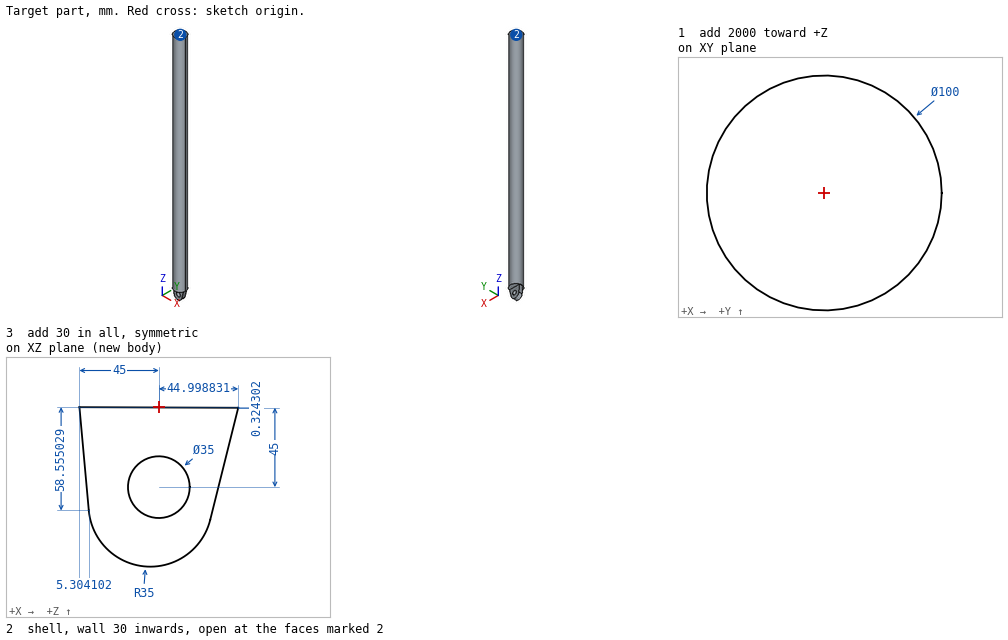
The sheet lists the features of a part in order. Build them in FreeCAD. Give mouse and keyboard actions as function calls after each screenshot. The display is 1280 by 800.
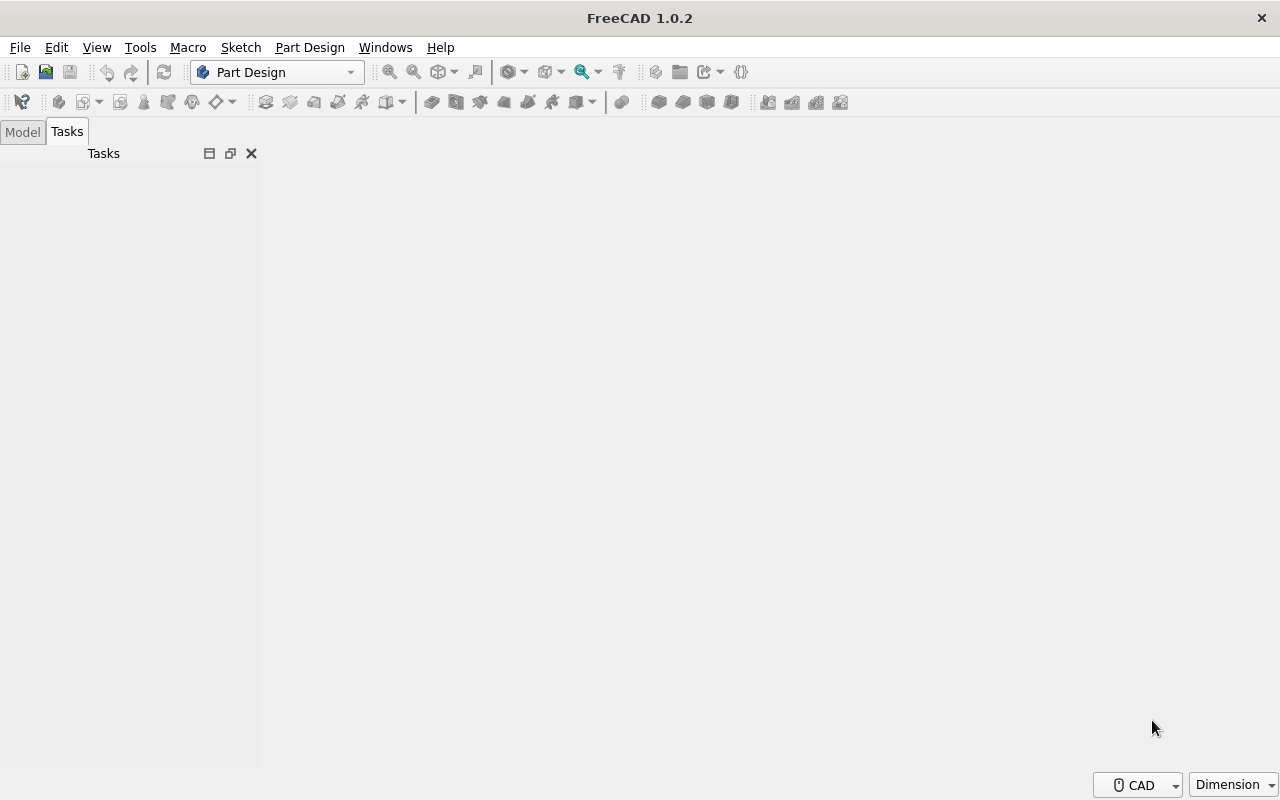
key(ctrl+n)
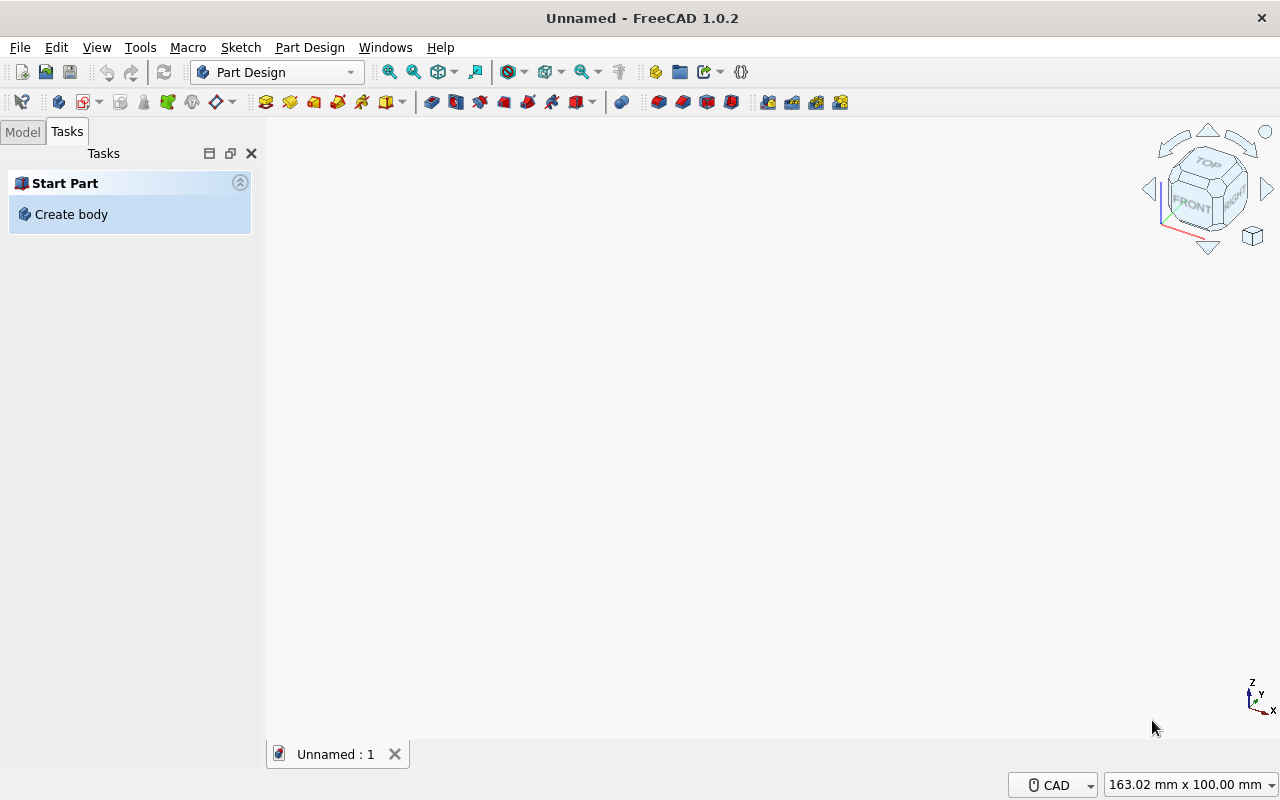
click(84, 102)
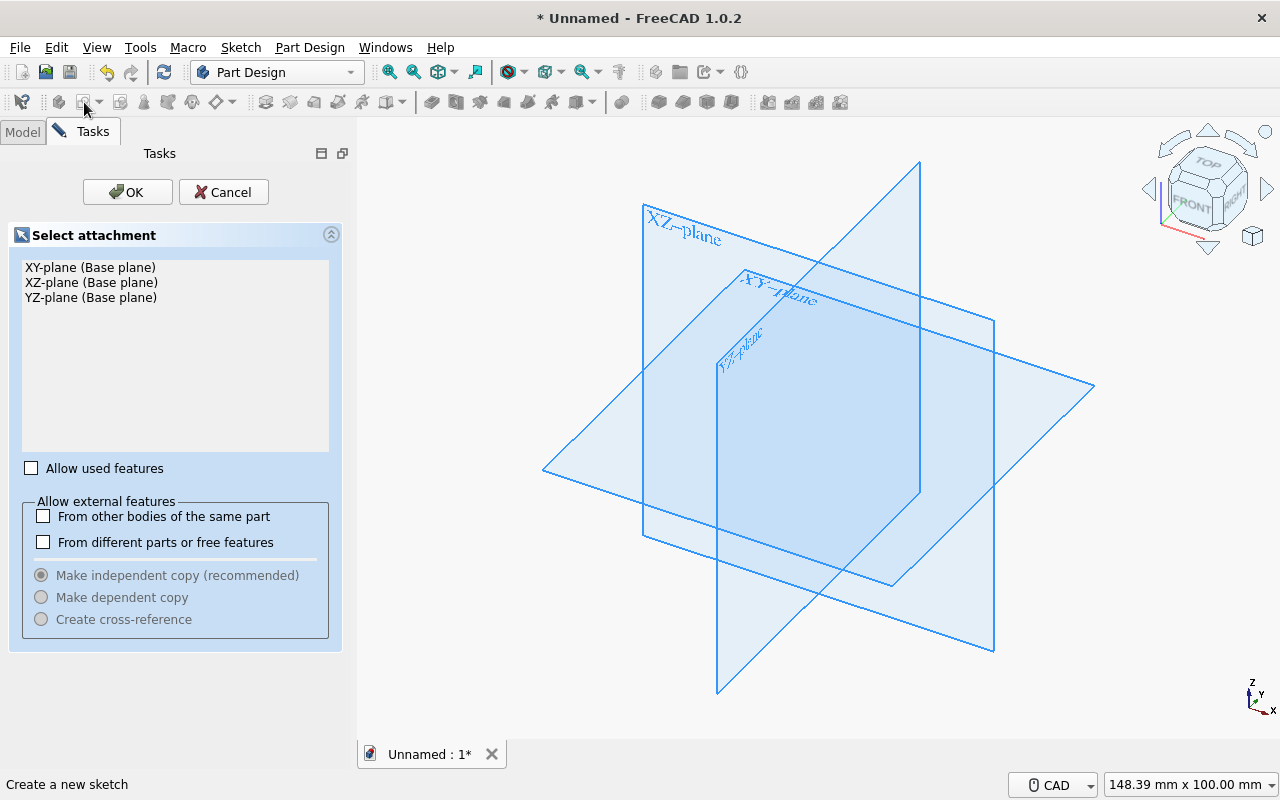
click(82, 268)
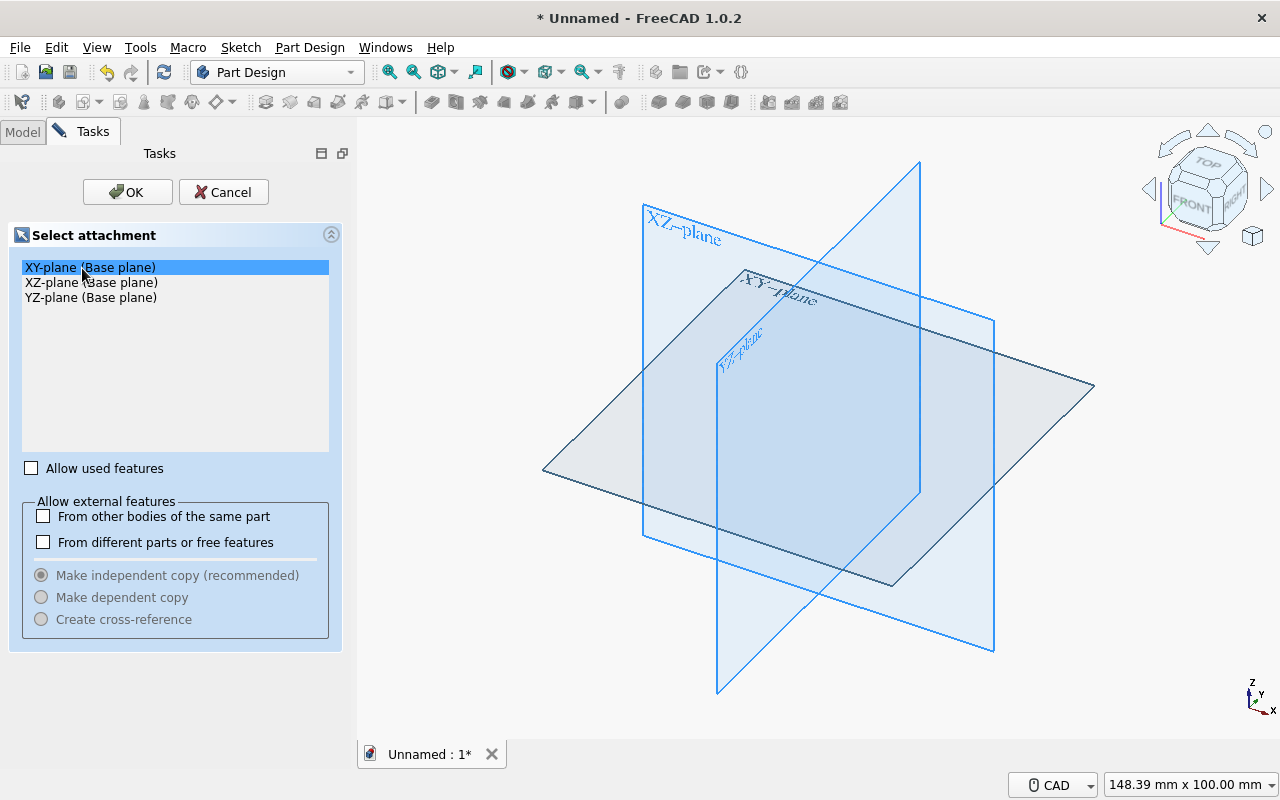
click(128, 192)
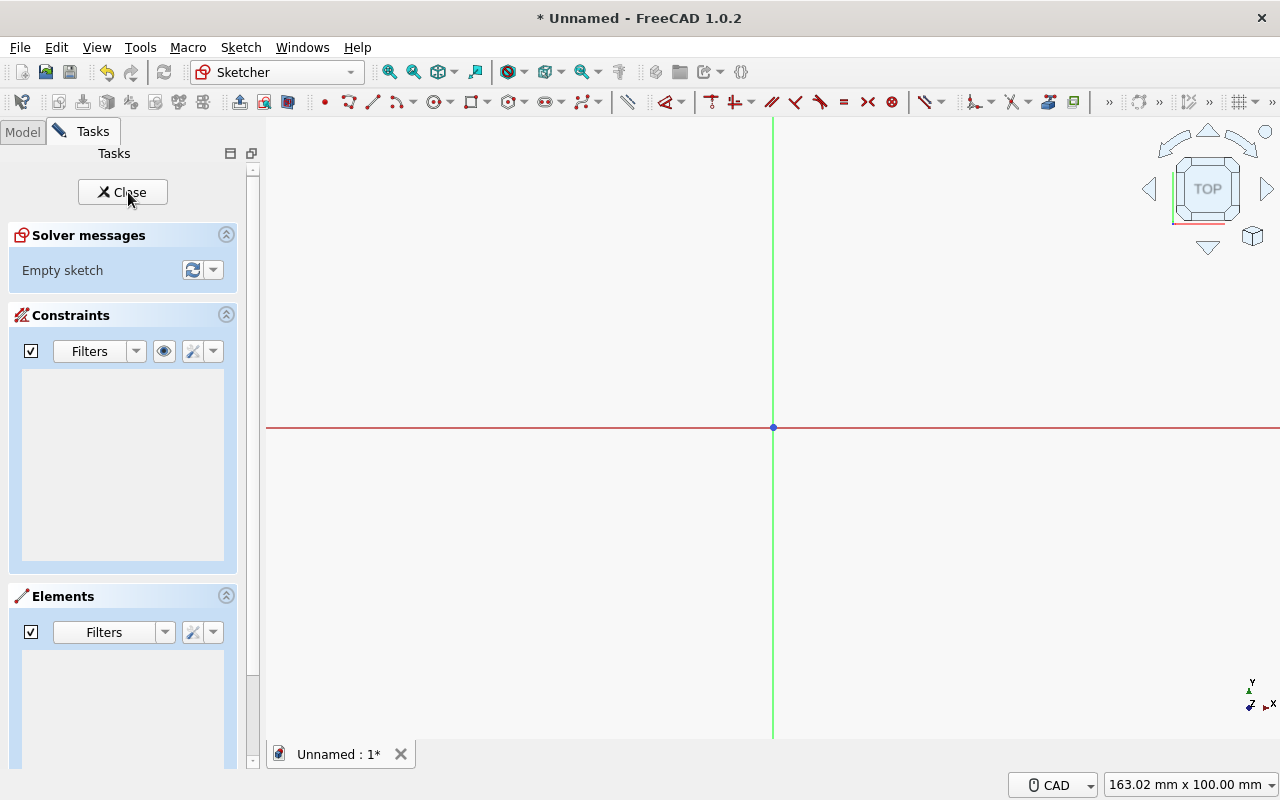
scroll(565, 428, down, 2)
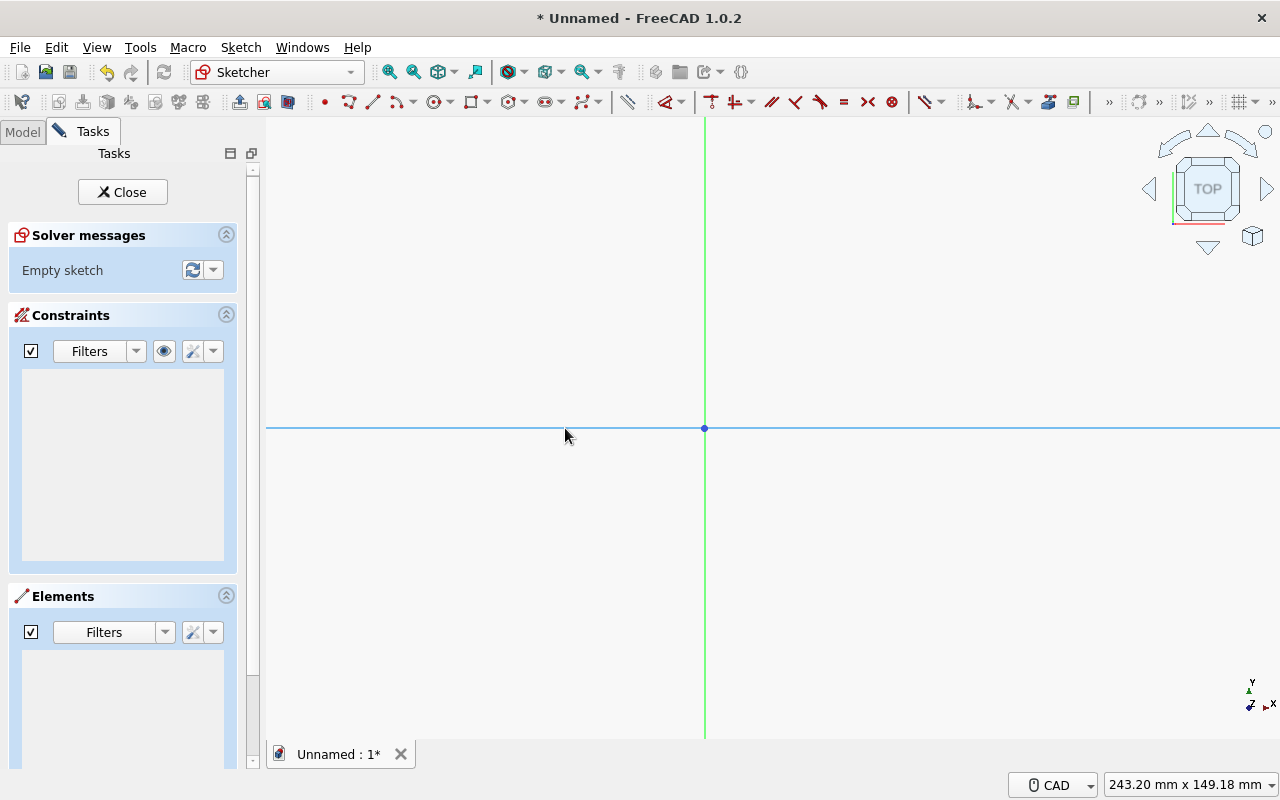
key(g)
key(c)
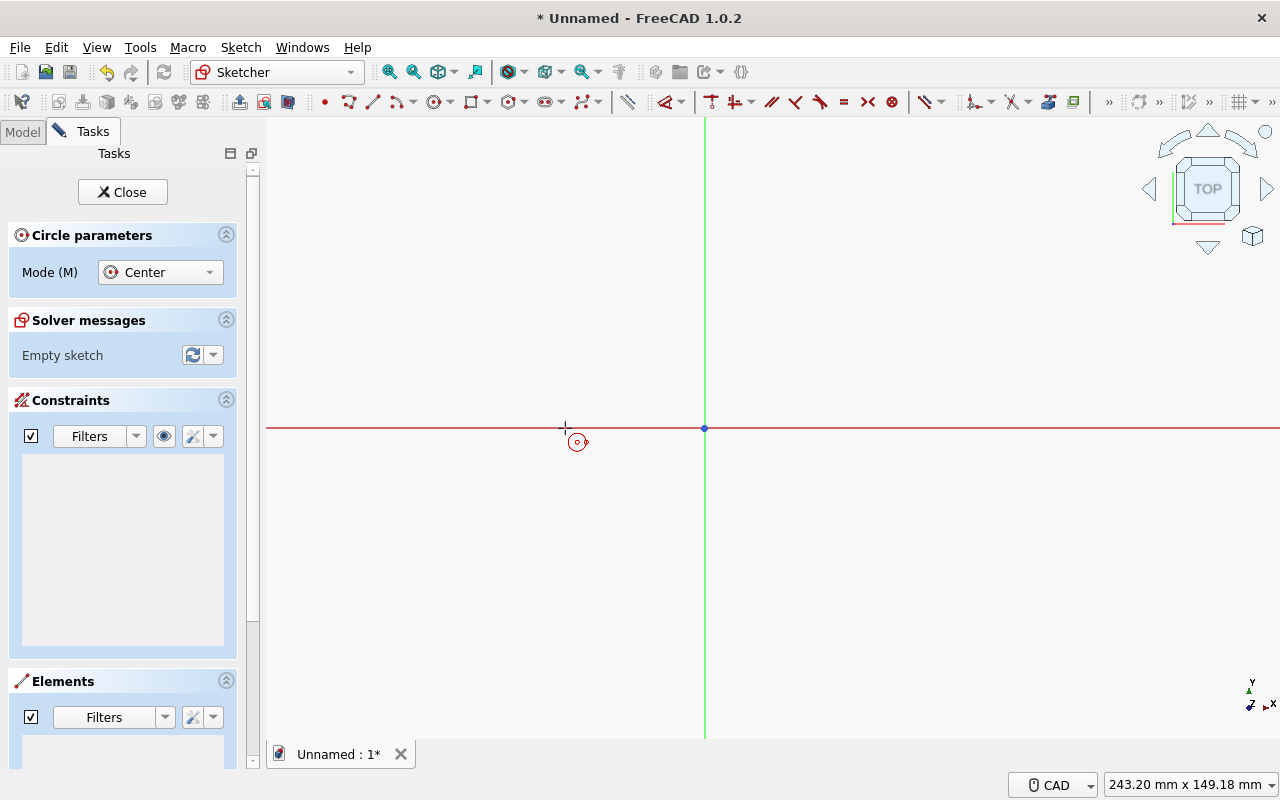
click(705, 428)
click(852, 281)
key(Escape)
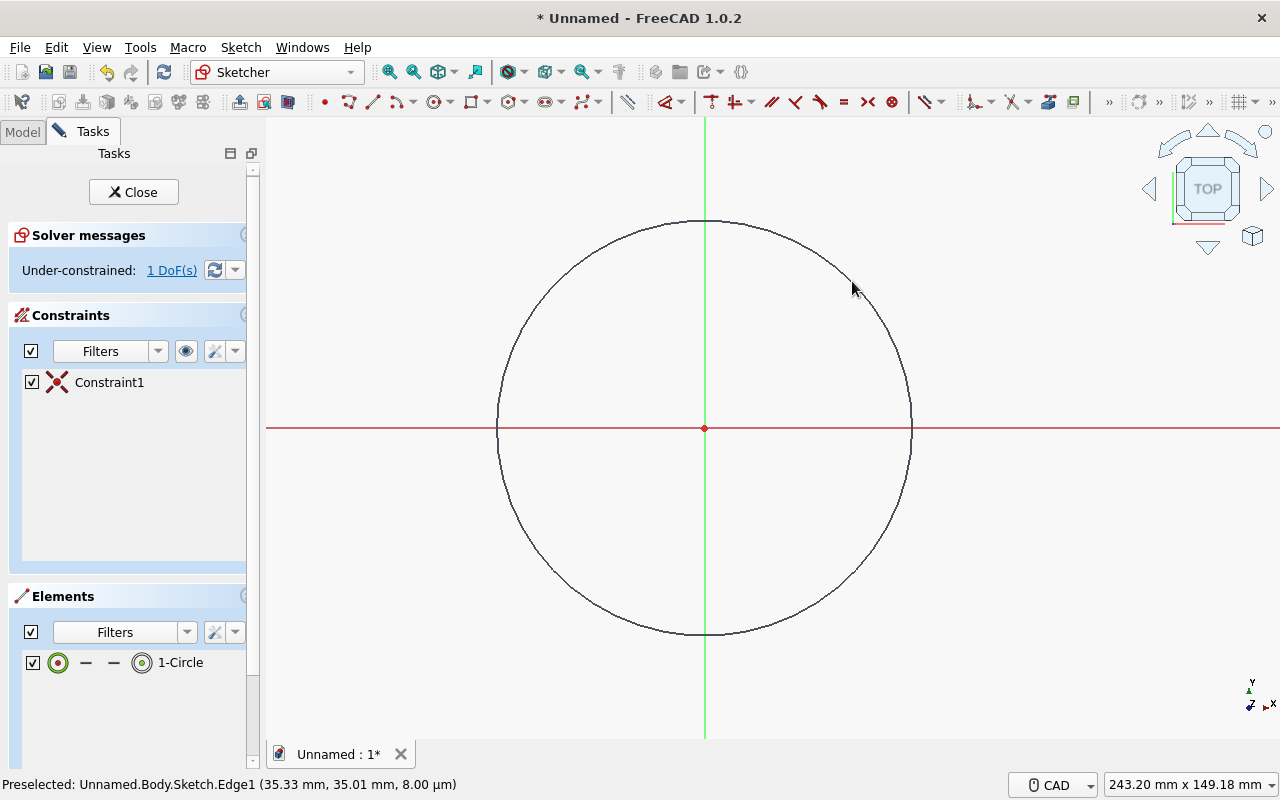
key(d)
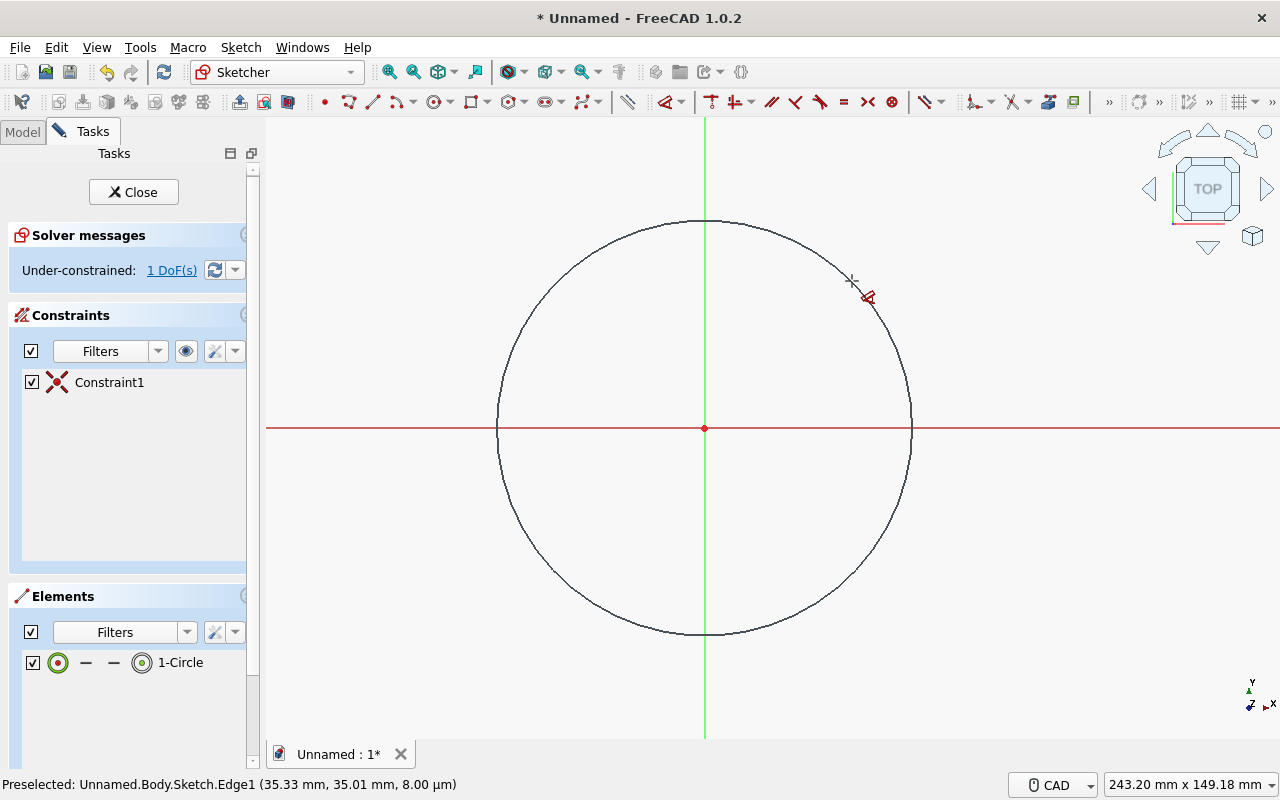
click(851, 281)
click(874, 258)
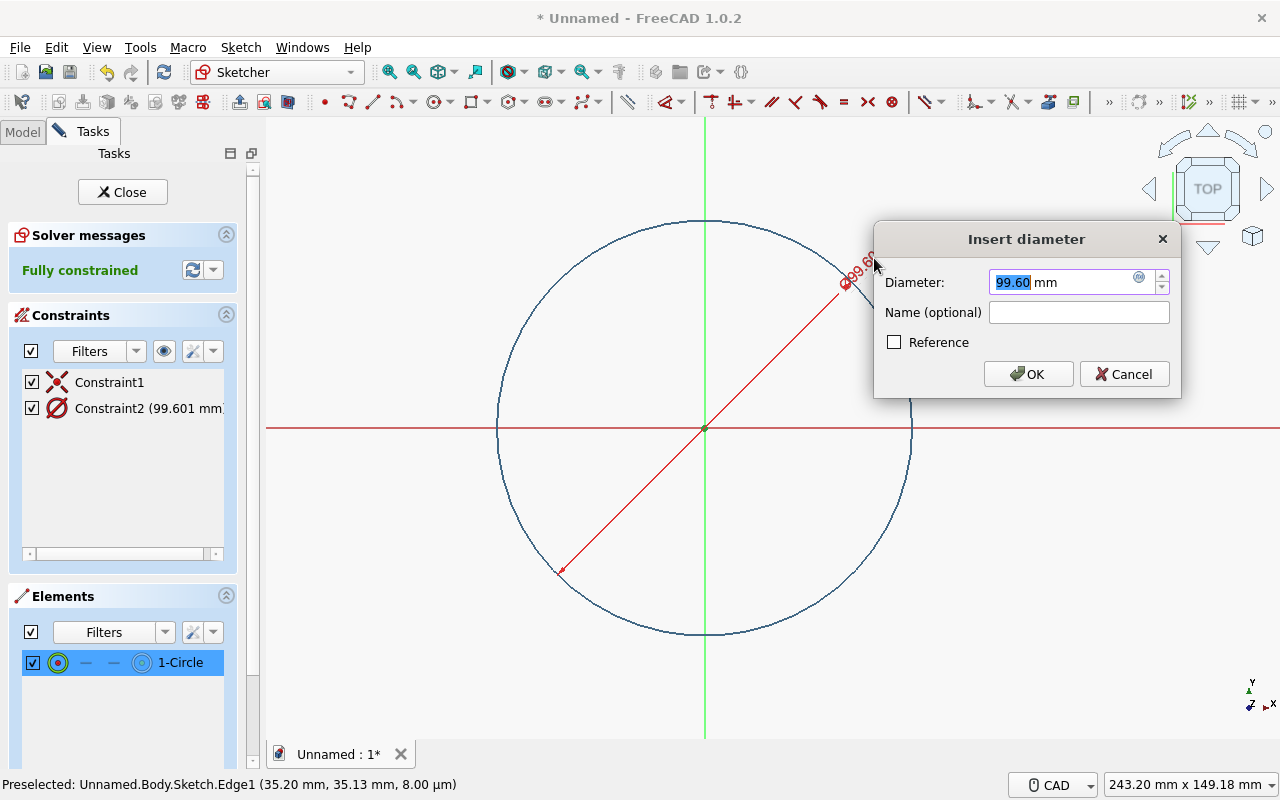
text(100)
key(Return)
key(Escape)